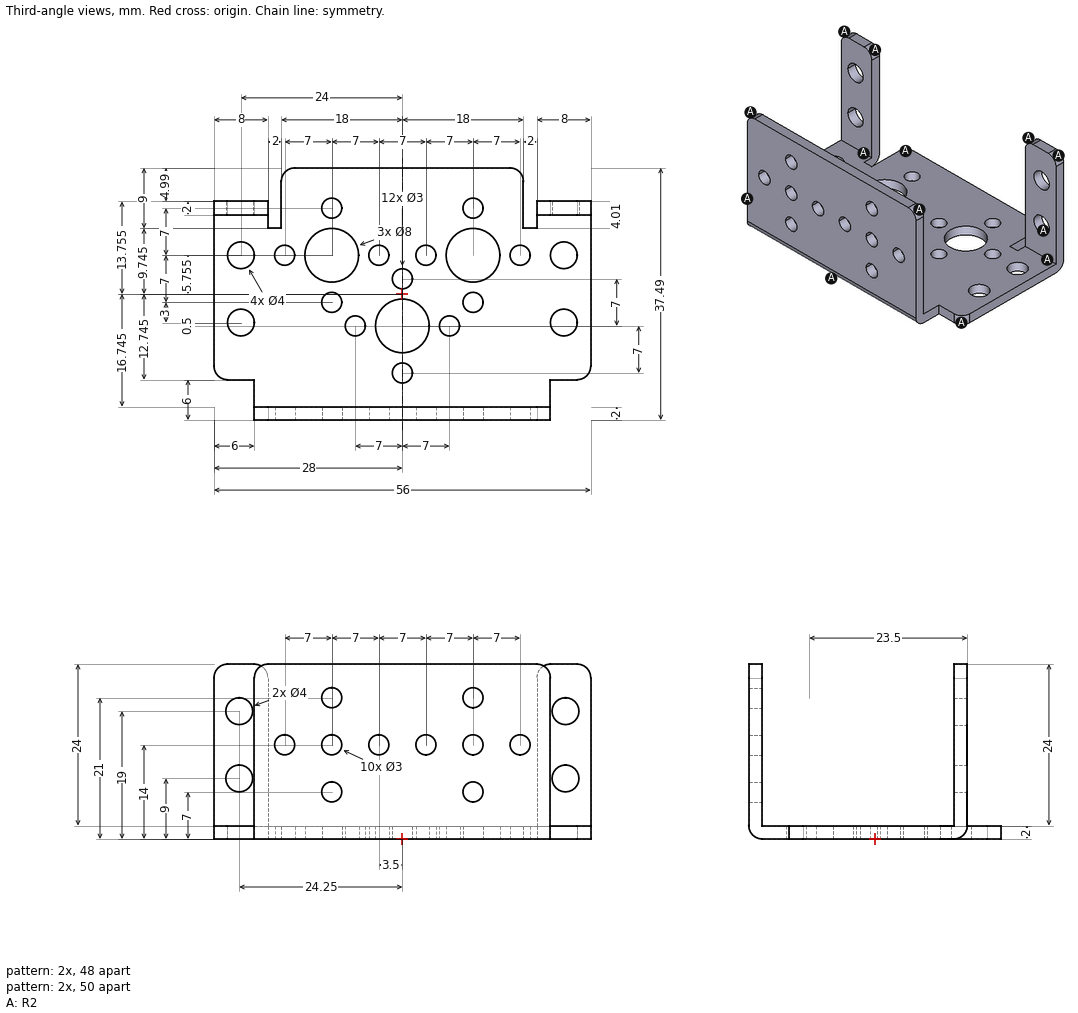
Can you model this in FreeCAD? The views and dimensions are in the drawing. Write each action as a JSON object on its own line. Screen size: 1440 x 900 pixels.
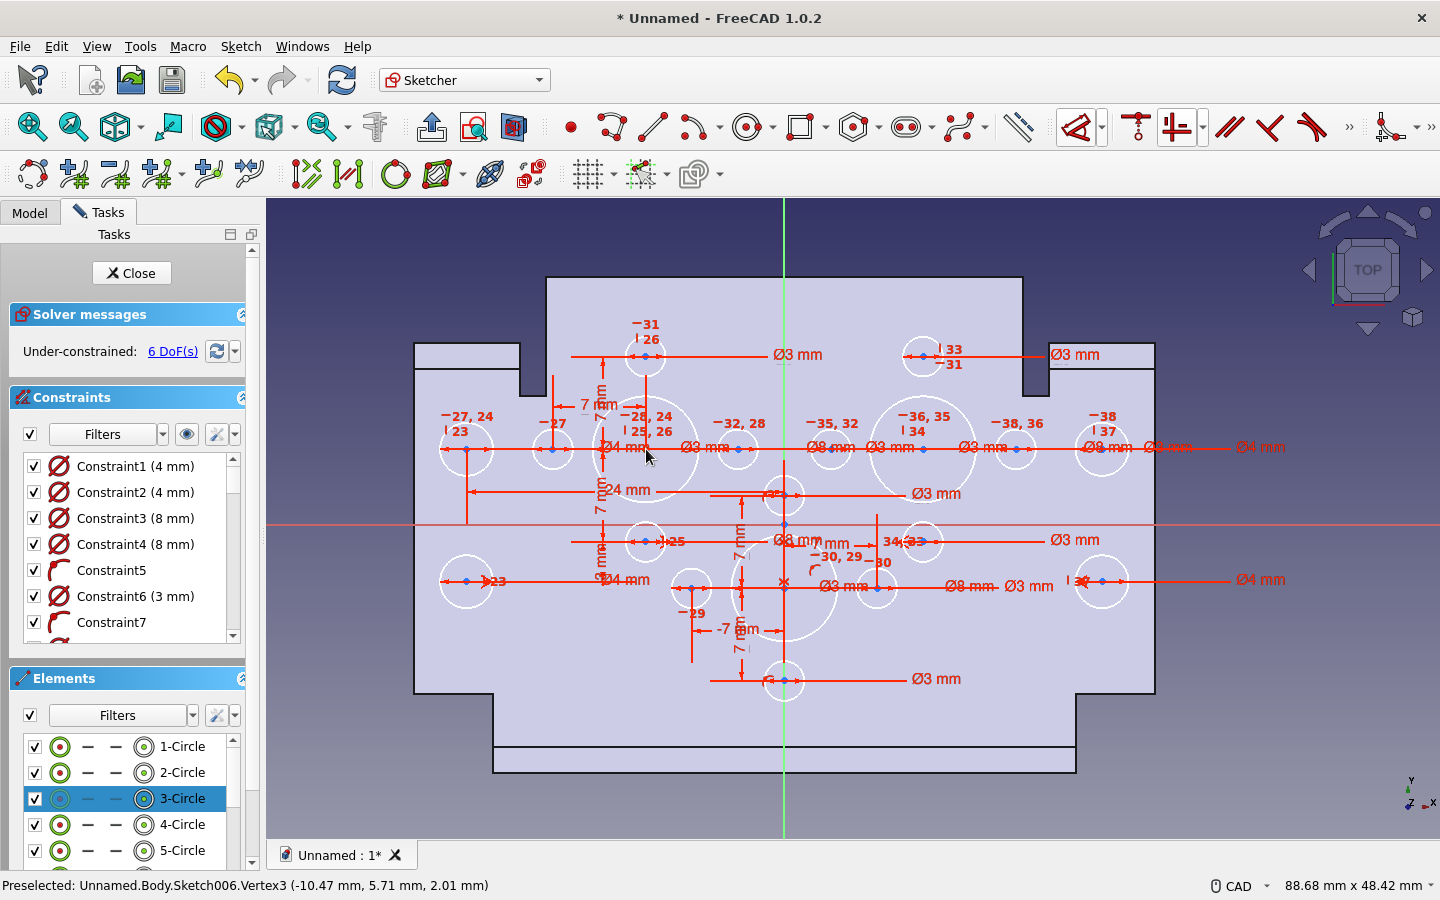
{"action": "left_click", "coordinate": [738, 449]}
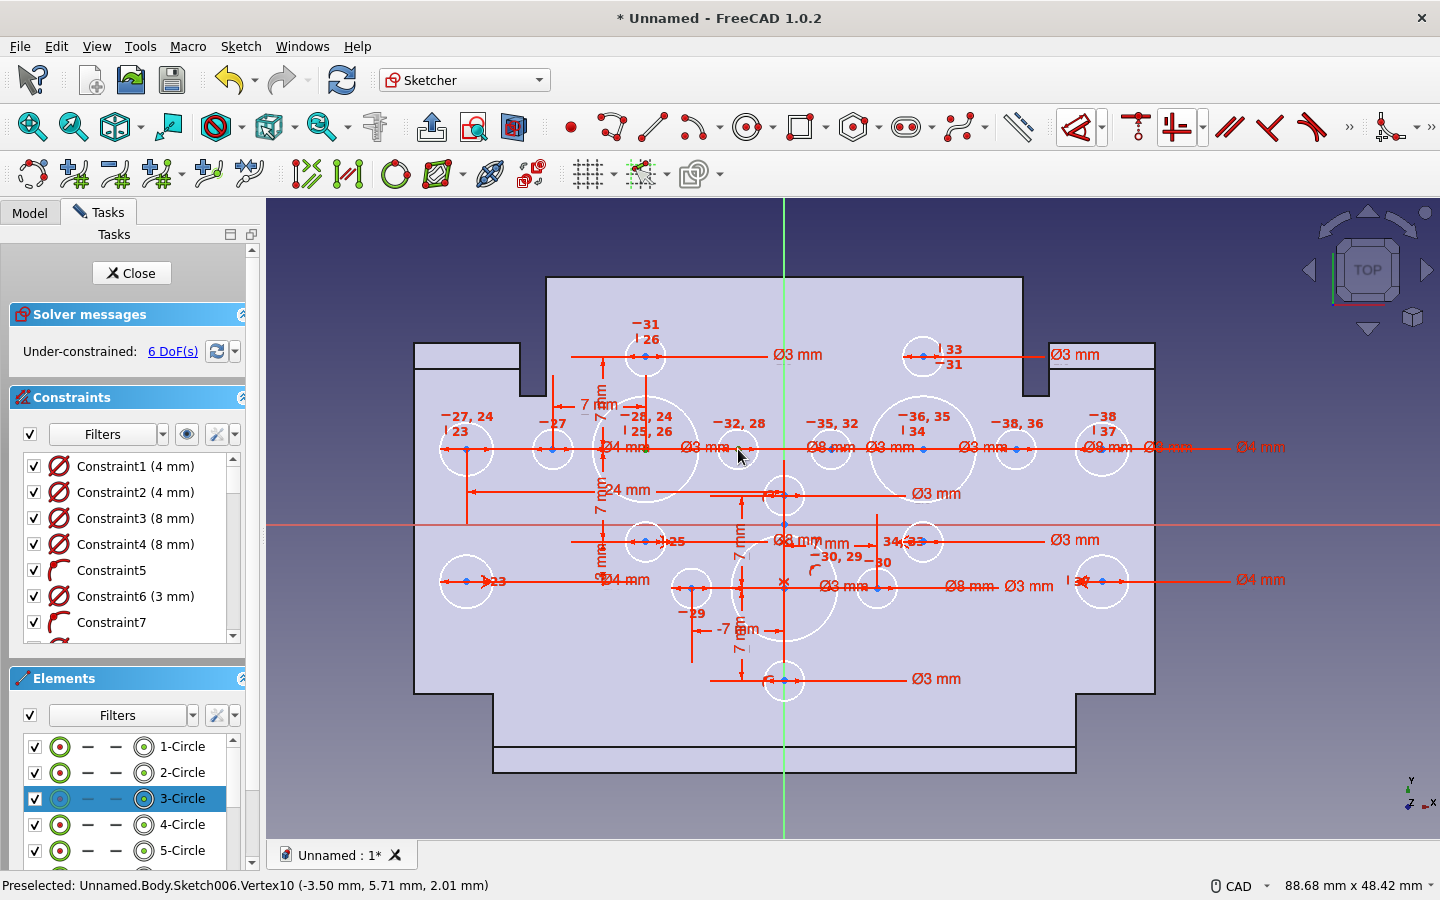
{"action": "key", "text": "l"}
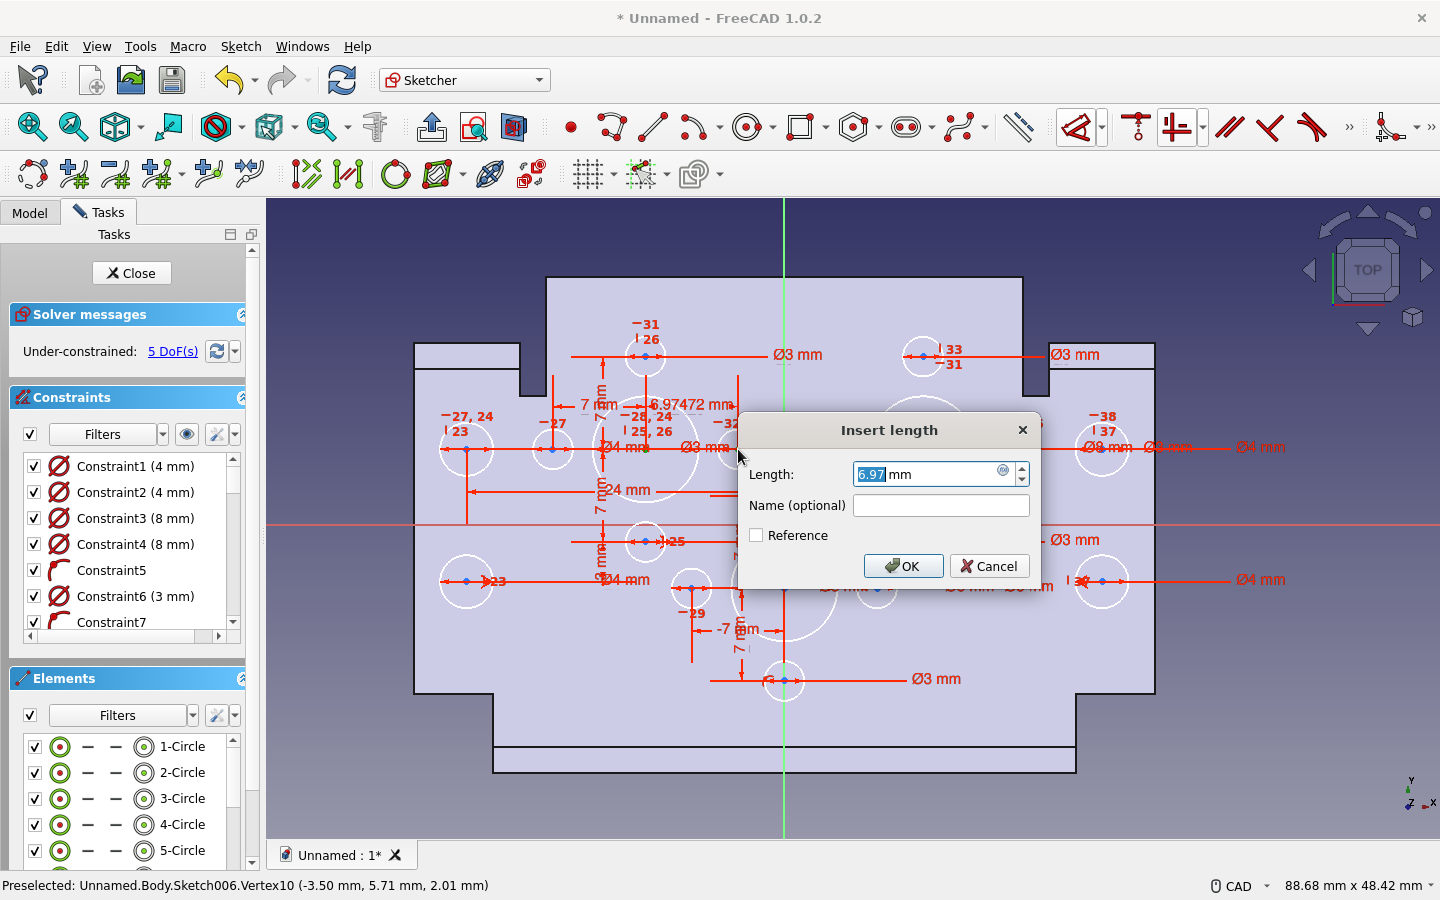
{"action": "type", "text": "7"}
{"action": "key", "text": "Return"}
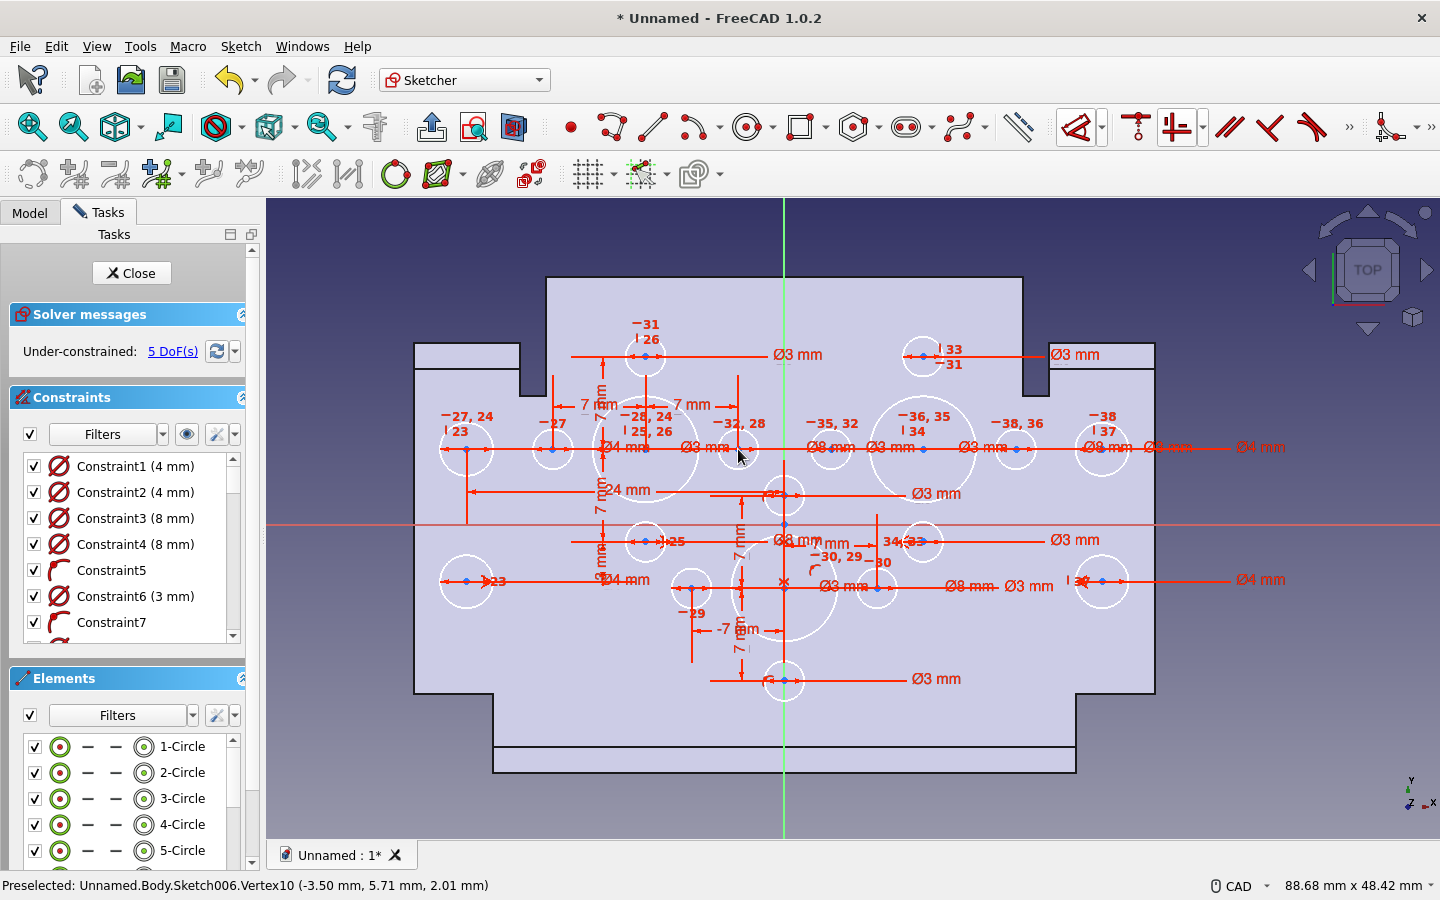
{"action": "left_click", "coordinate": [738, 449]}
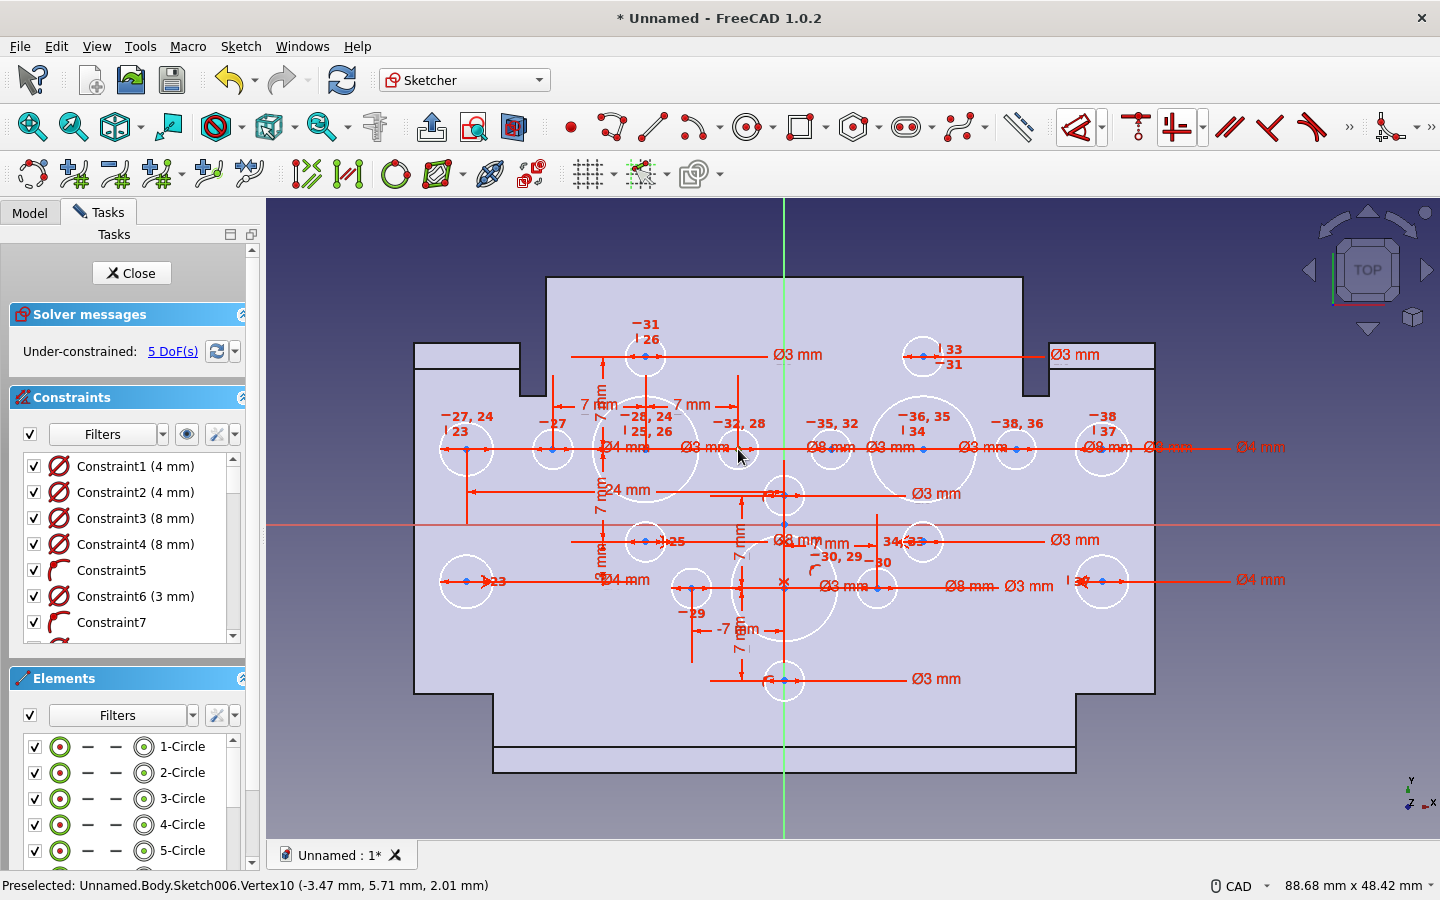
{"action": "left_click", "coordinate": [831, 449]}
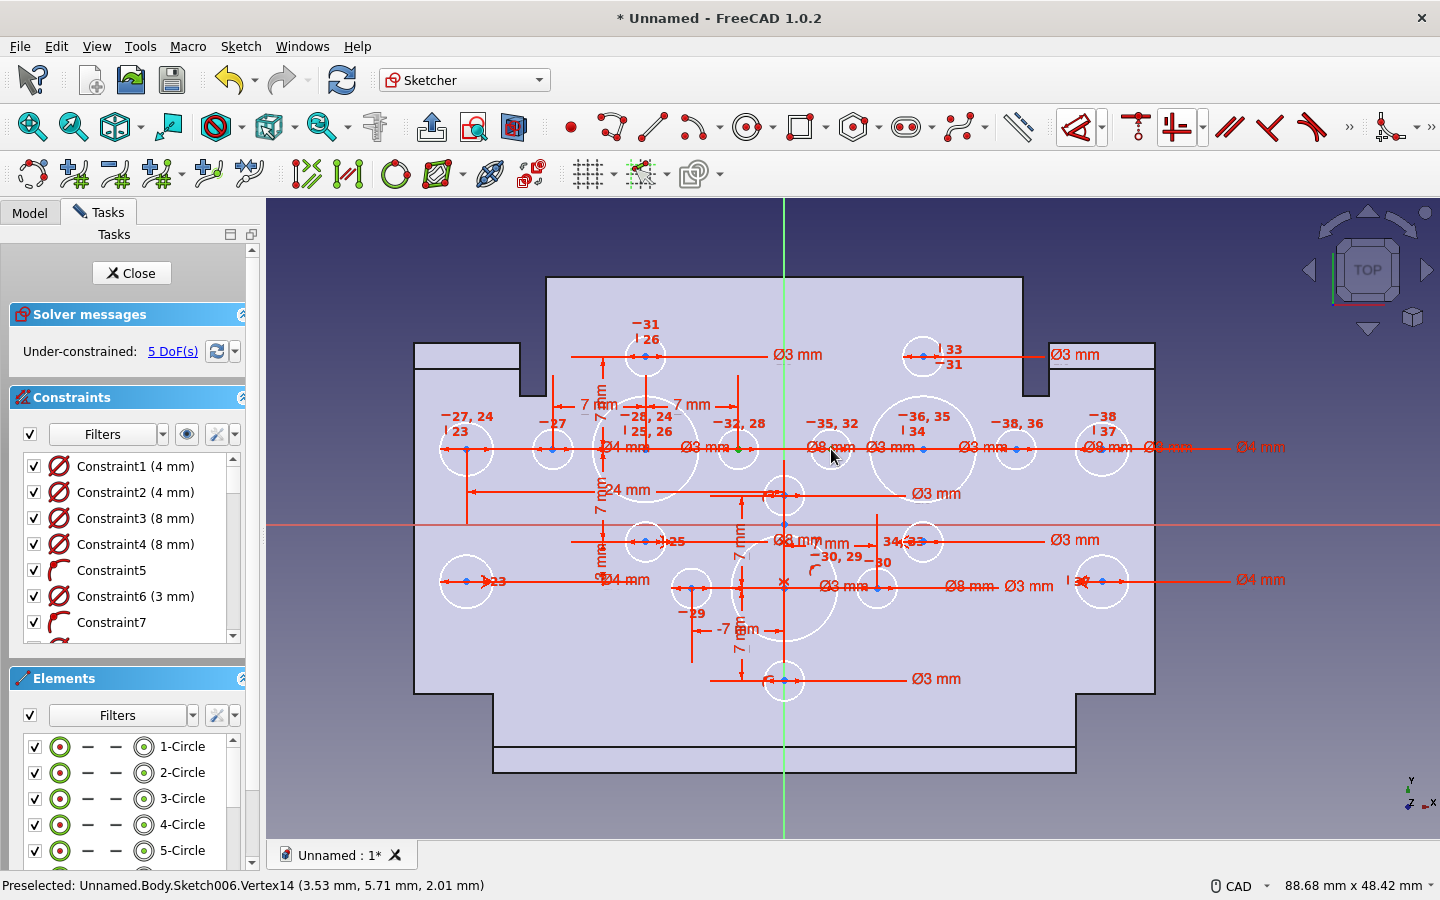
{"action": "left_click", "coordinate": [1102, 128]}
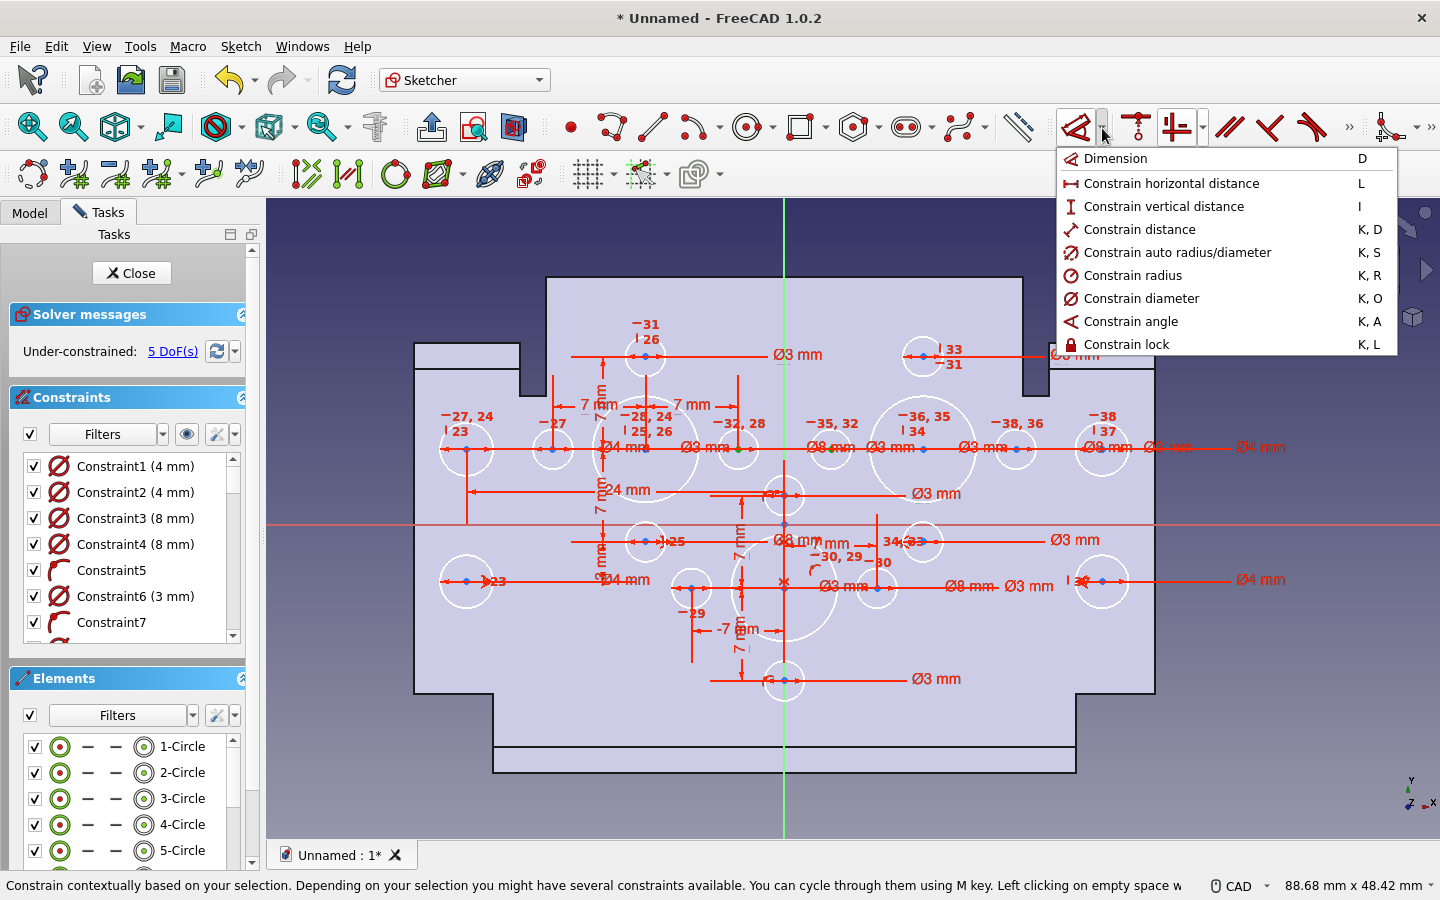
{"action": "left_click", "coordinate": [1227, 184]}